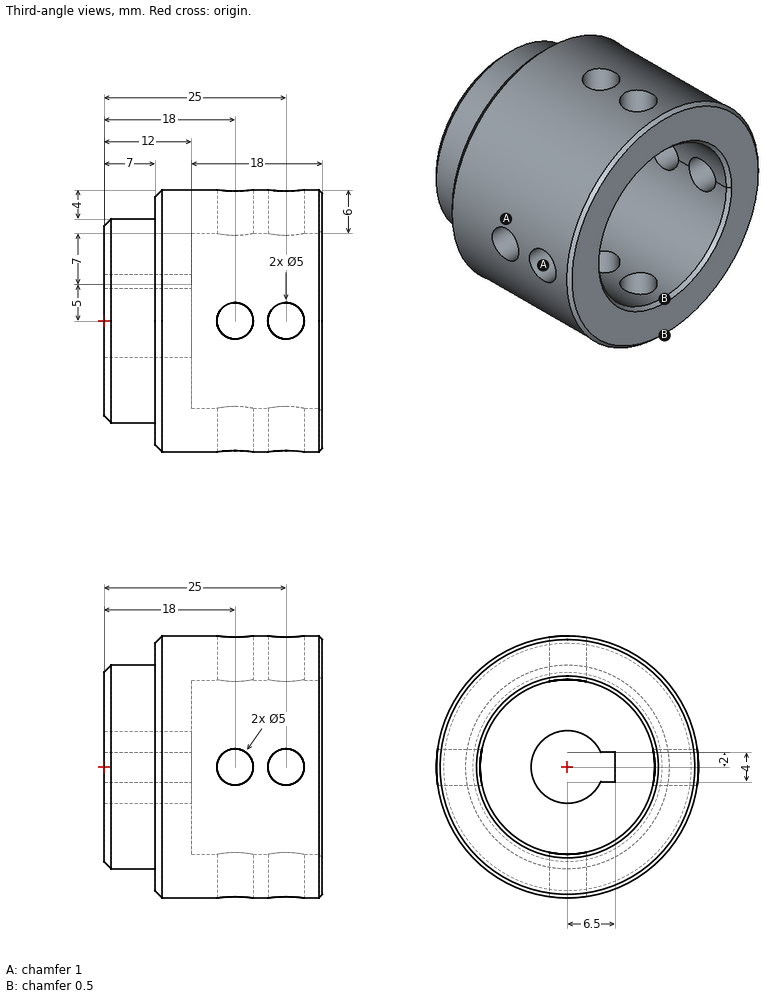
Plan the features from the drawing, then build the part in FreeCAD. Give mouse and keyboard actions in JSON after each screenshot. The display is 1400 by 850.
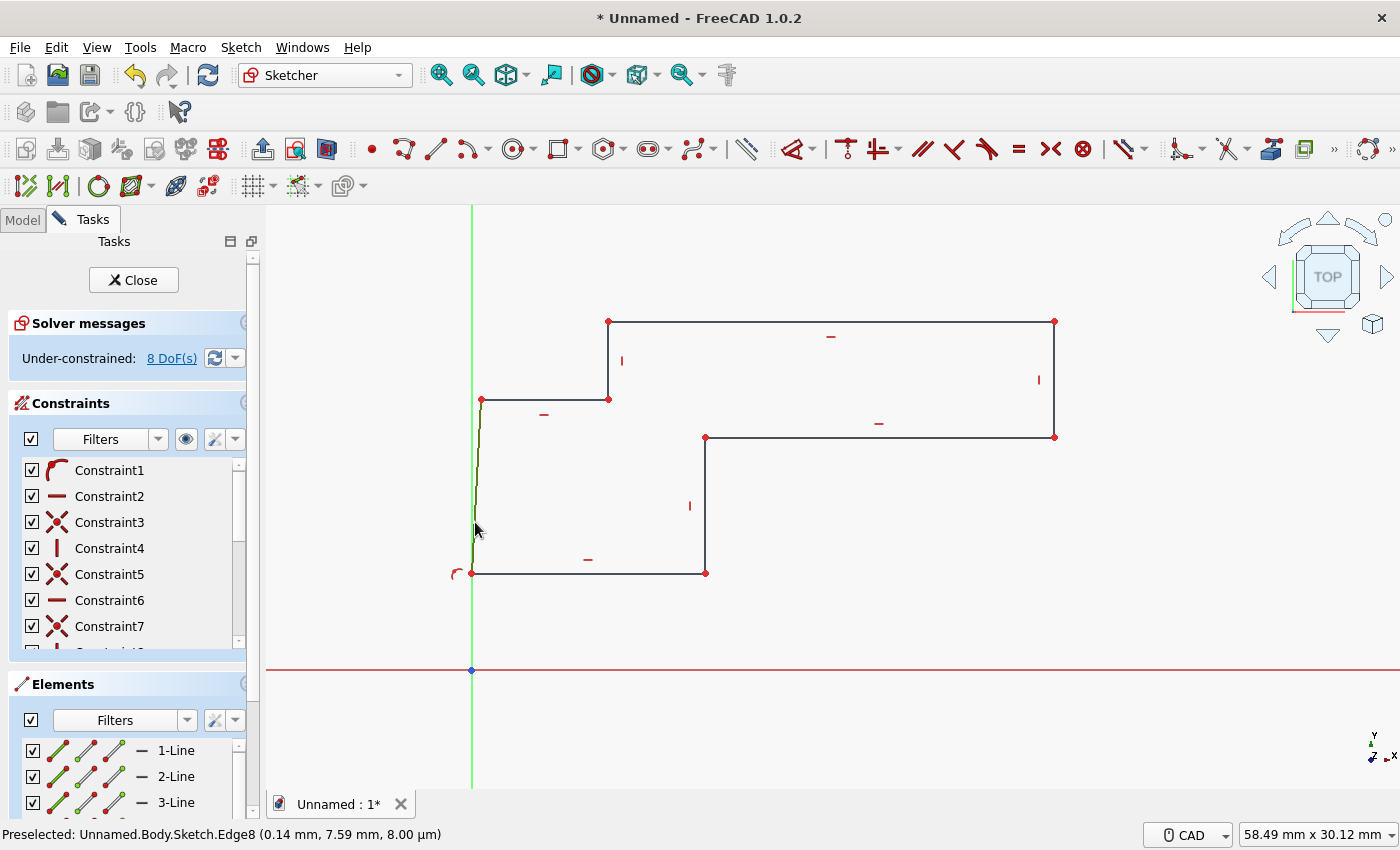
{"action": "key", "text": "v"}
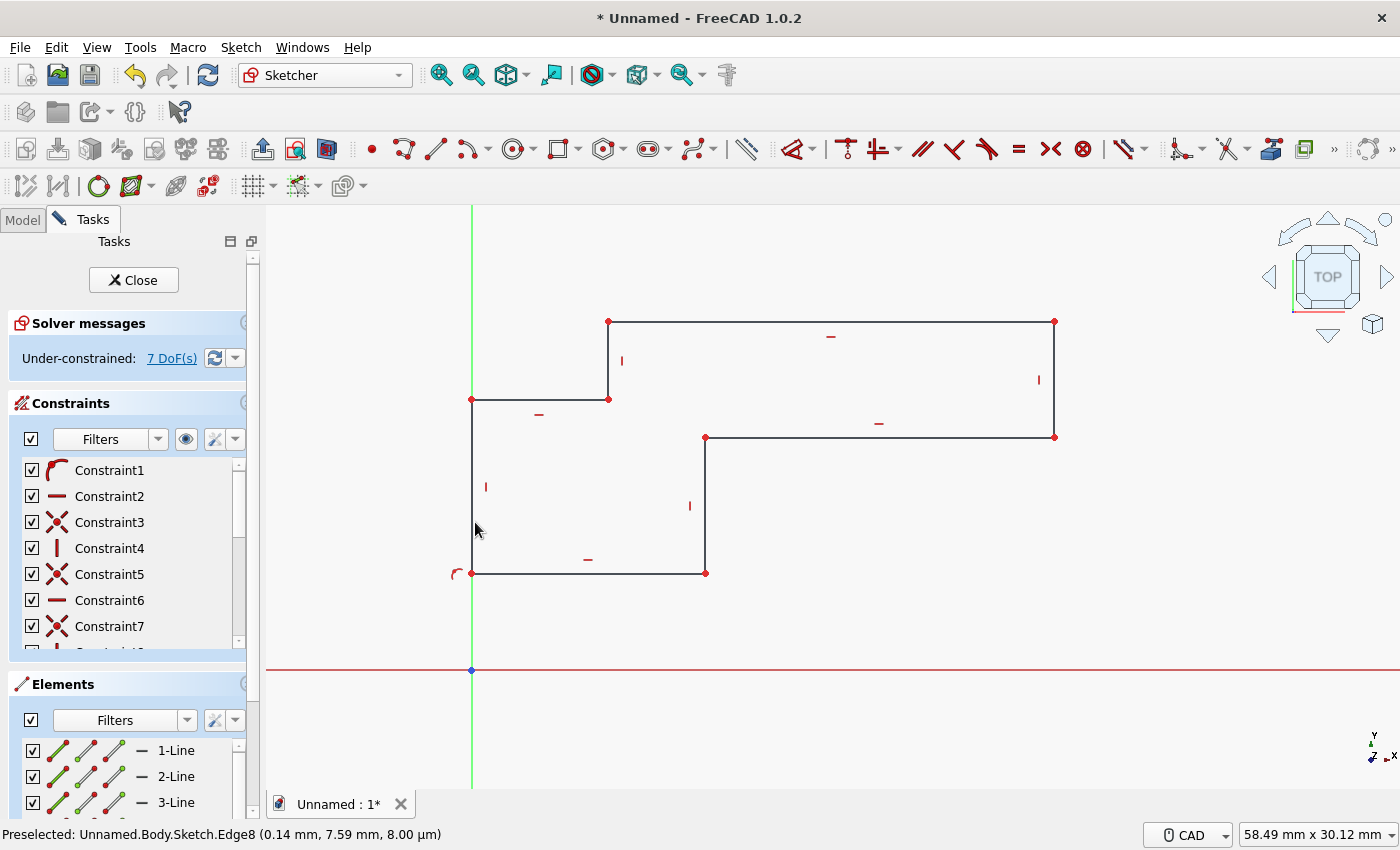
{"action": "left_click", "coordinate": [705, 533]}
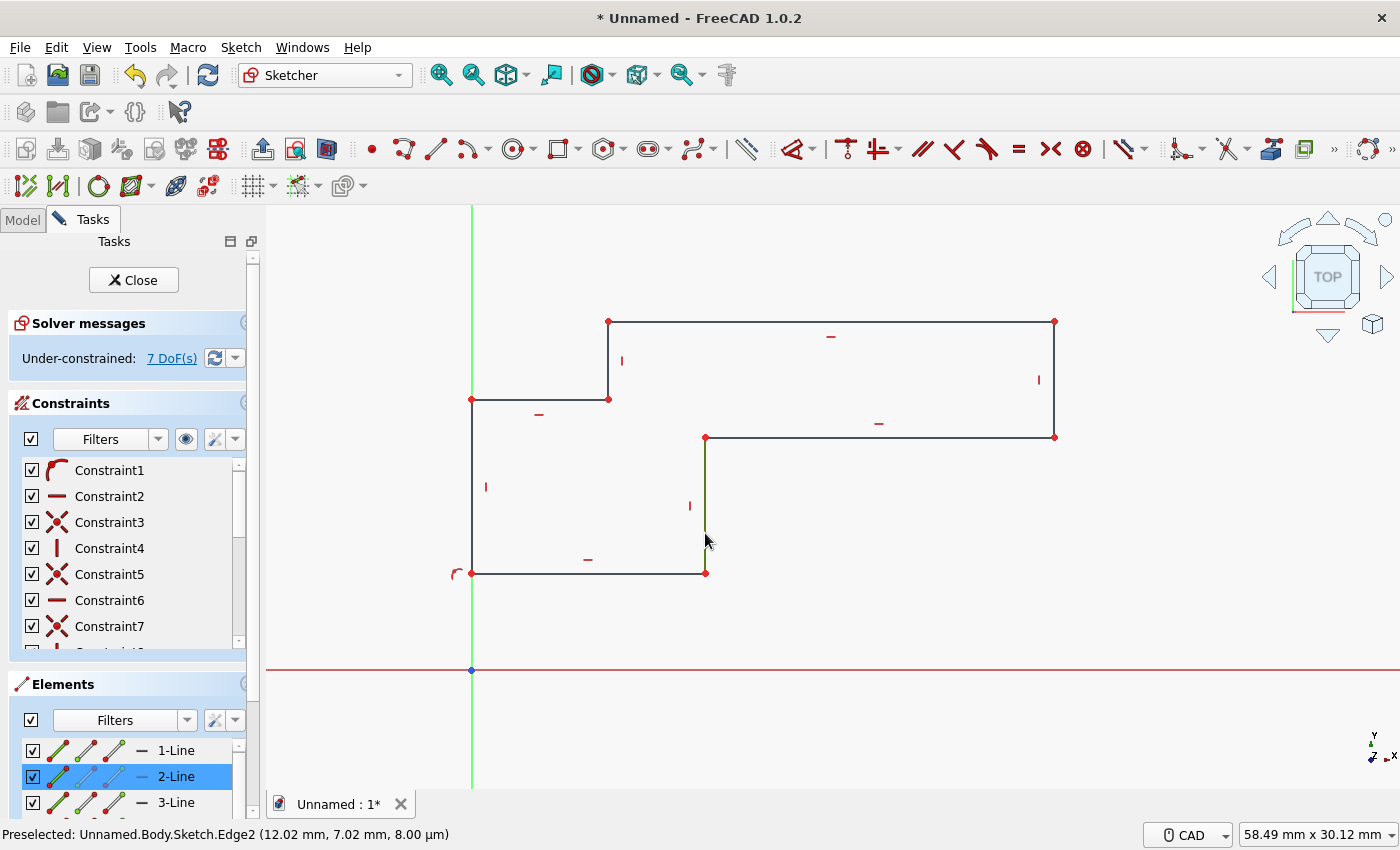
{"action": "key", "text": "i"}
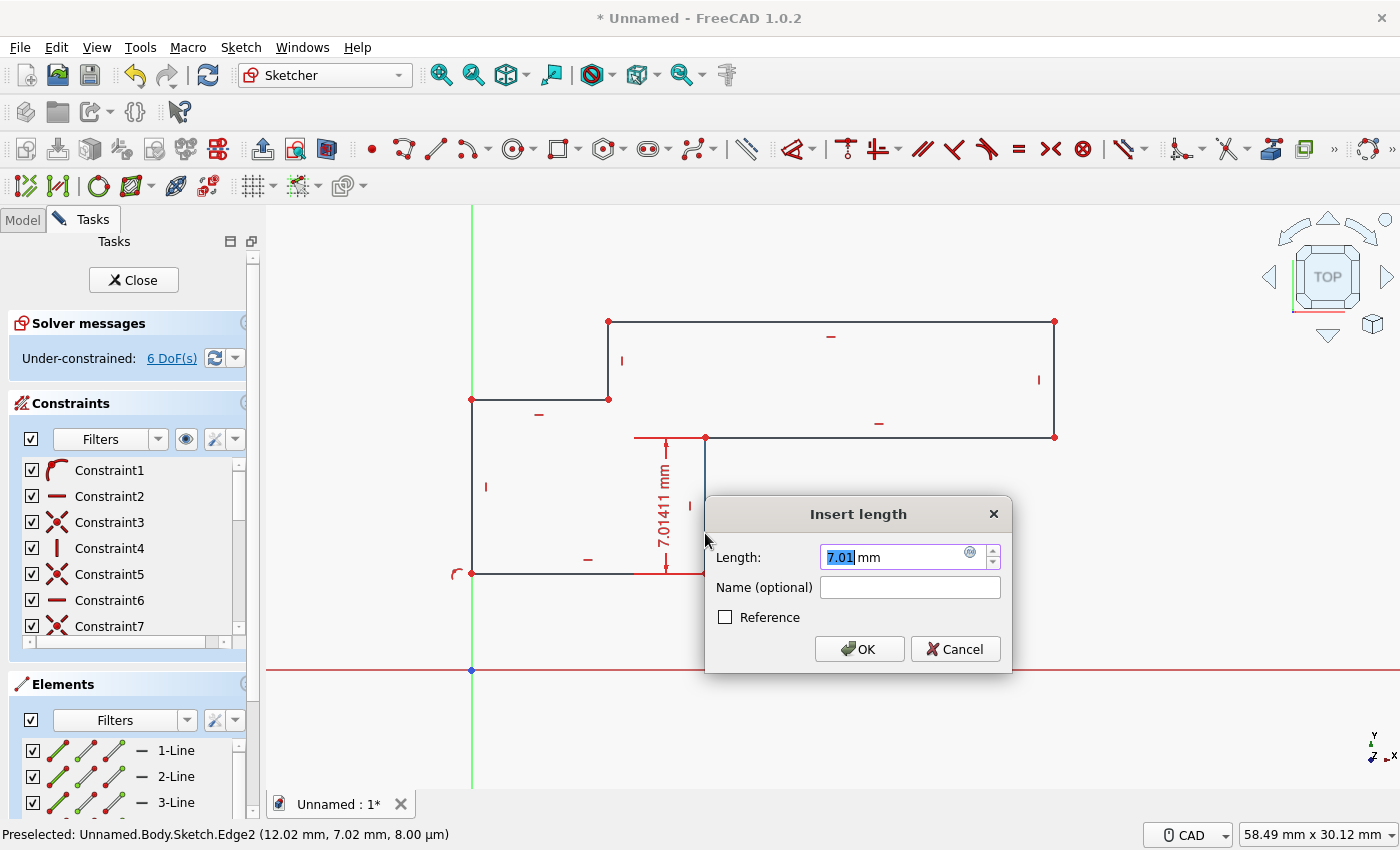
{"action": "type", "text": "7"}
{"action": "key", "text": "Return"}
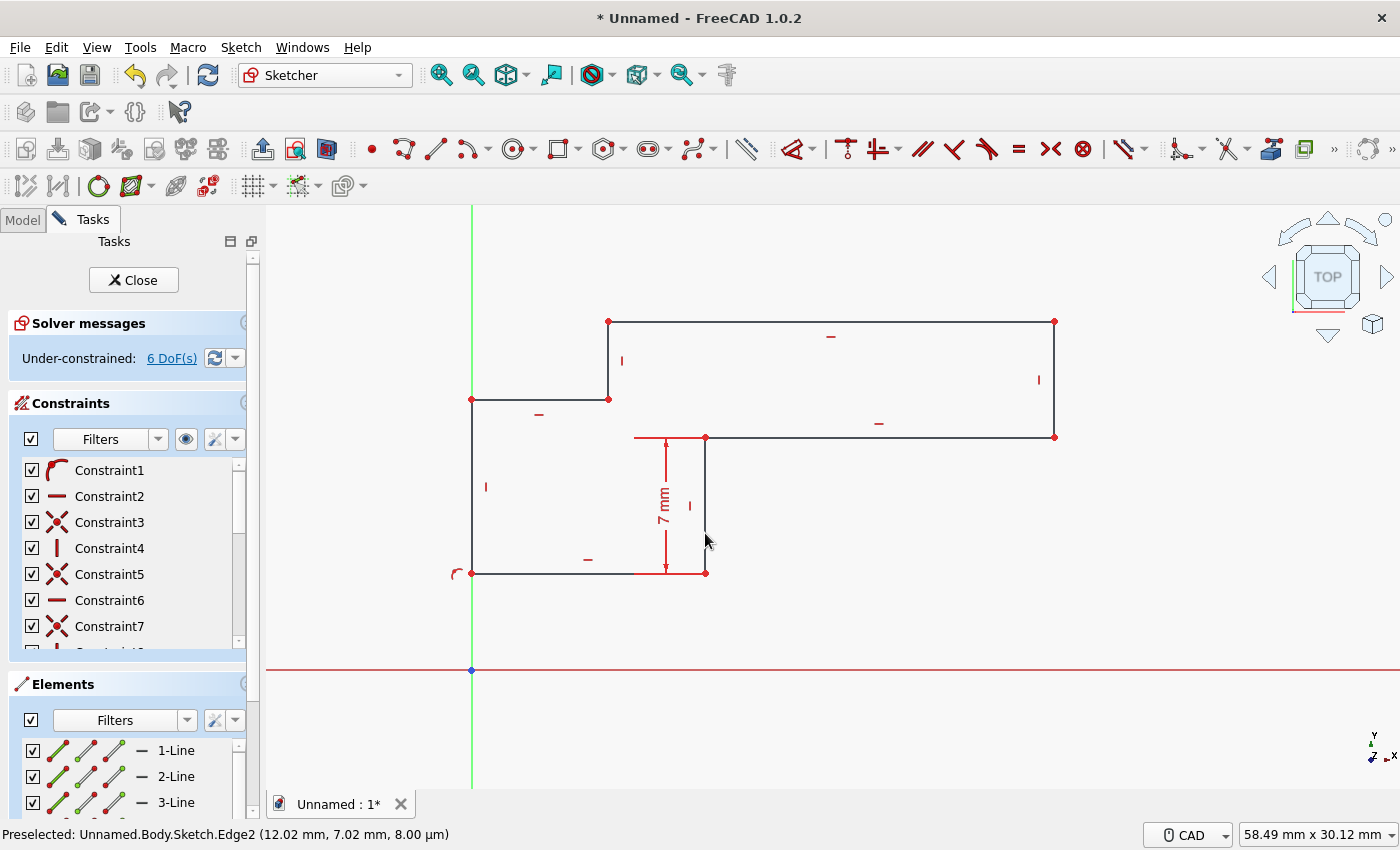
{"action": "left_click", "coordinate": [1054, 403]}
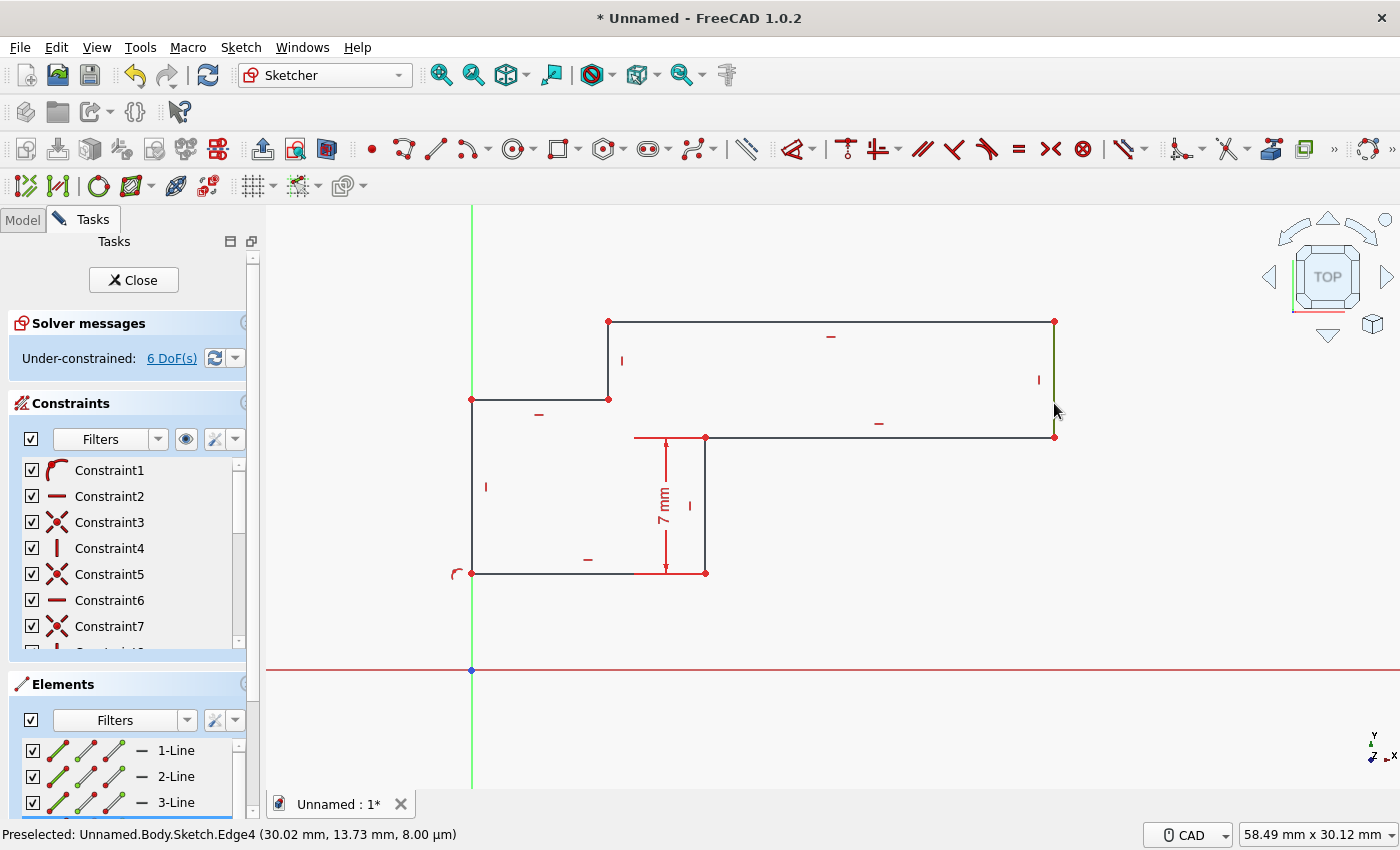
{"action": "left_click", "coordinate": [814, 150]}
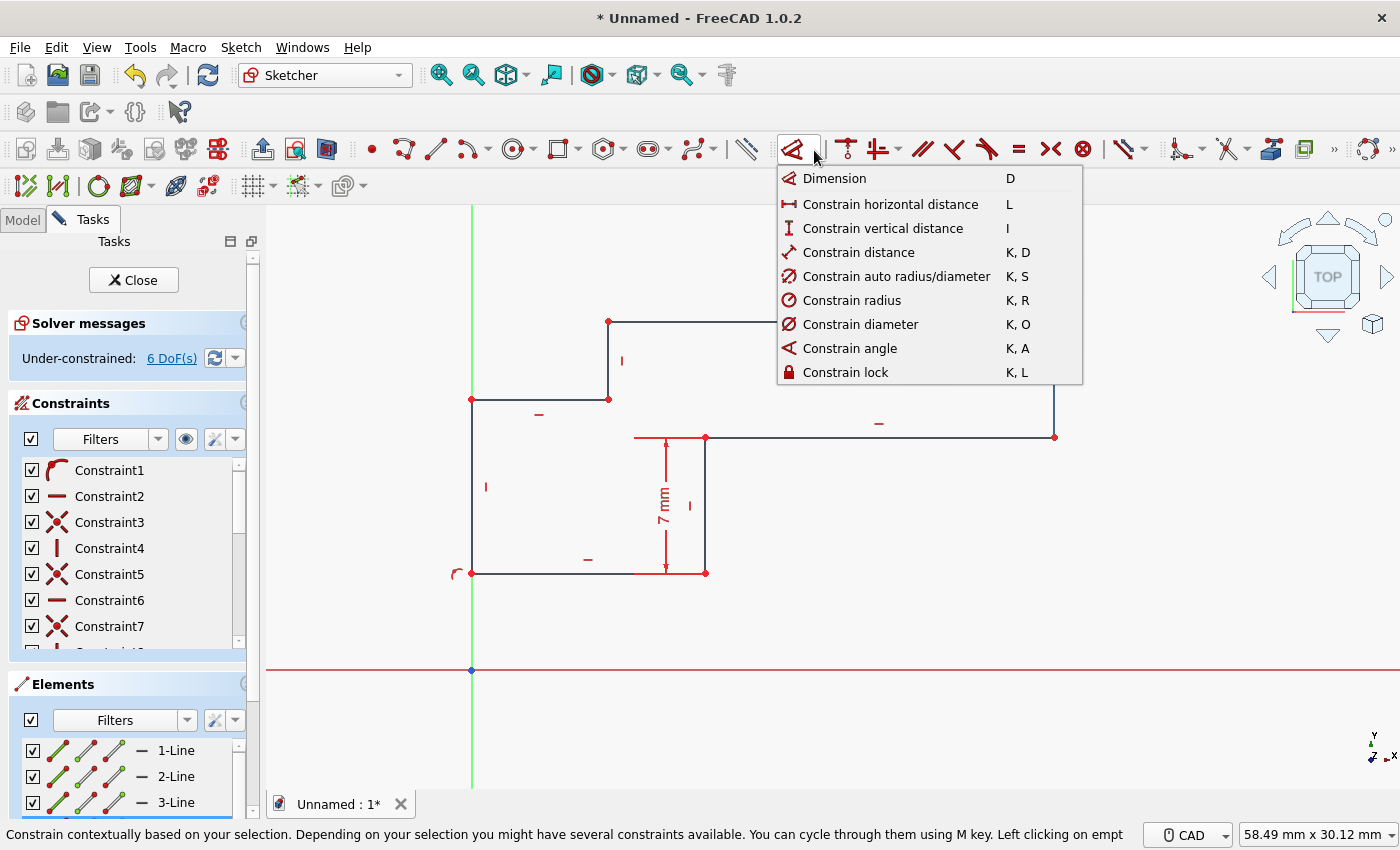
{"action": "left_click", "coordinate": [930, 228]}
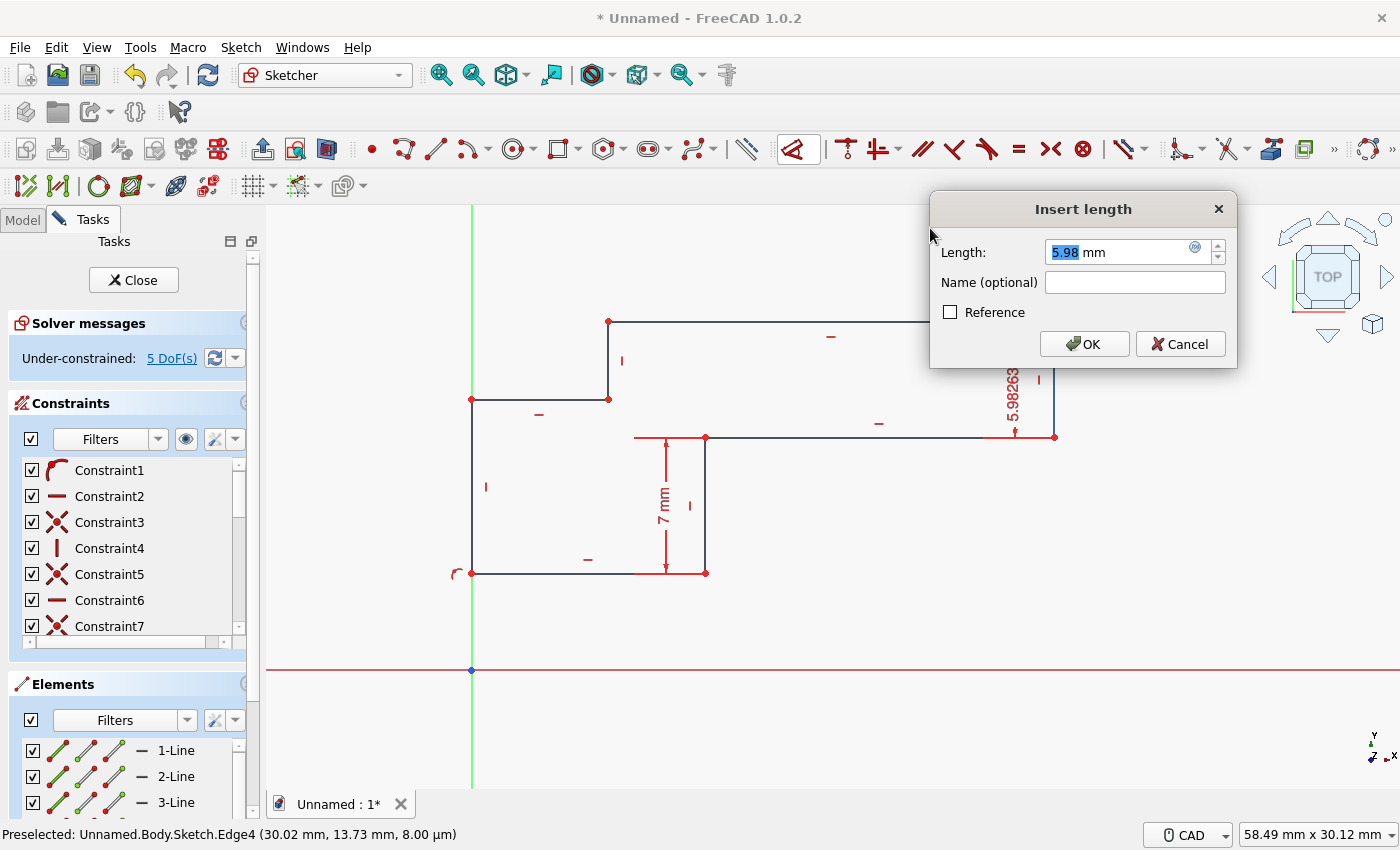
{"action": "type", "text": "6"}
{"action": "key", "text": "Return"}